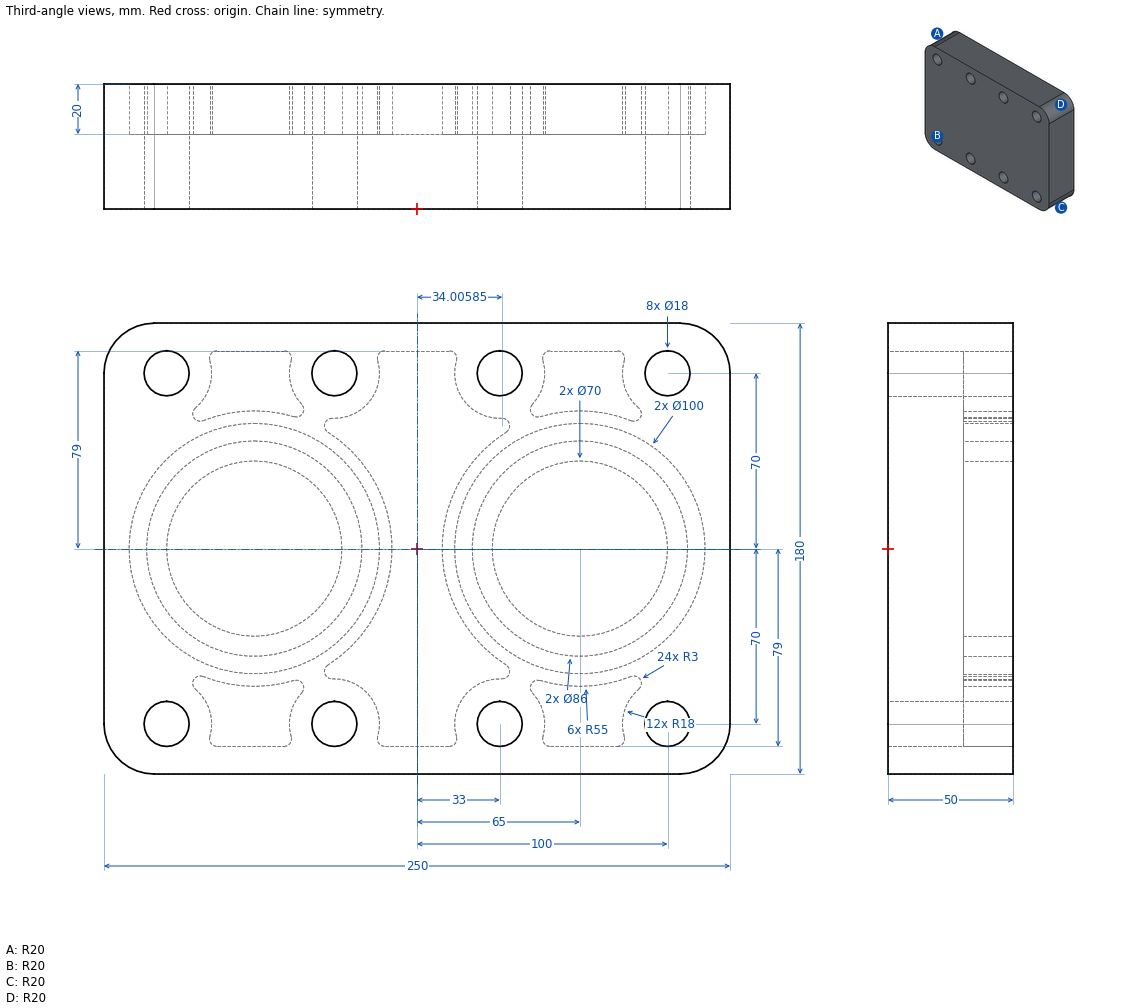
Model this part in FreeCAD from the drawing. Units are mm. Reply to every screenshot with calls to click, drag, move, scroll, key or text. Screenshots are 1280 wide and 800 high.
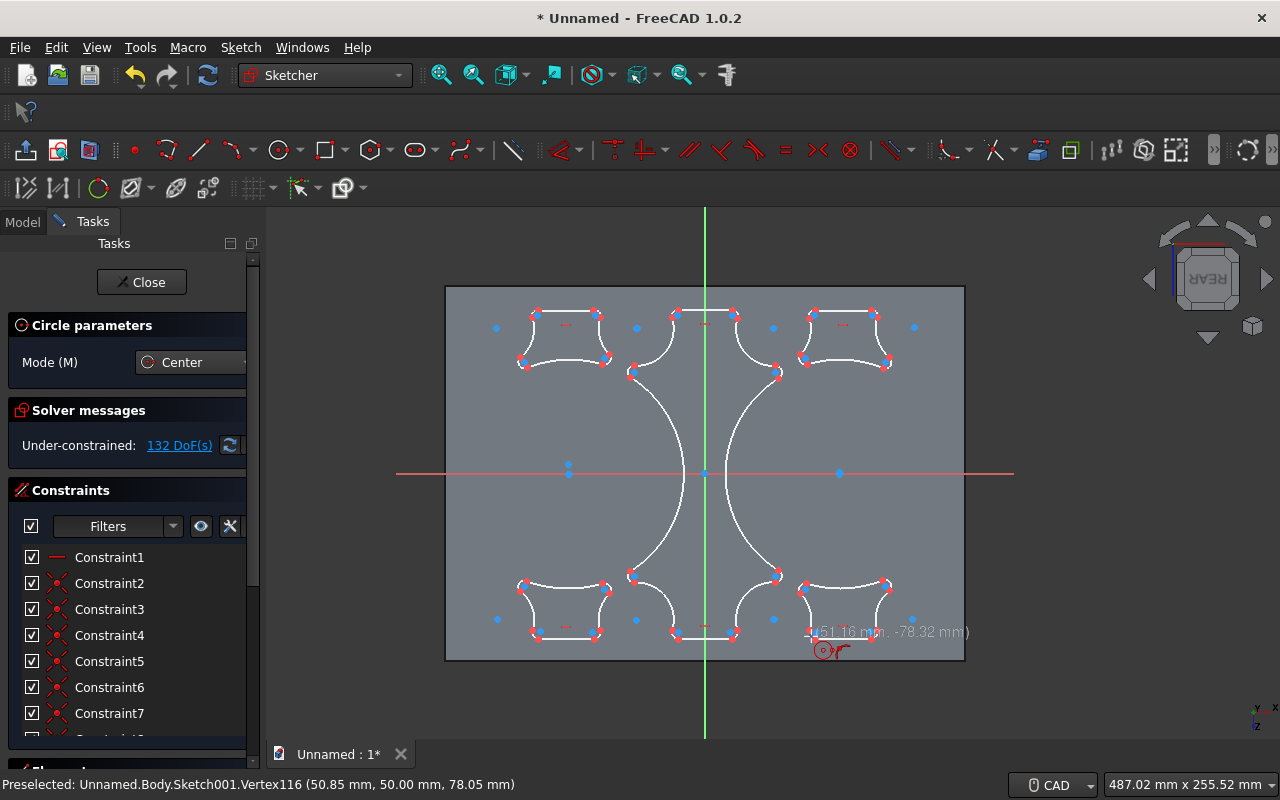
click(840, 474)
move(914, 400)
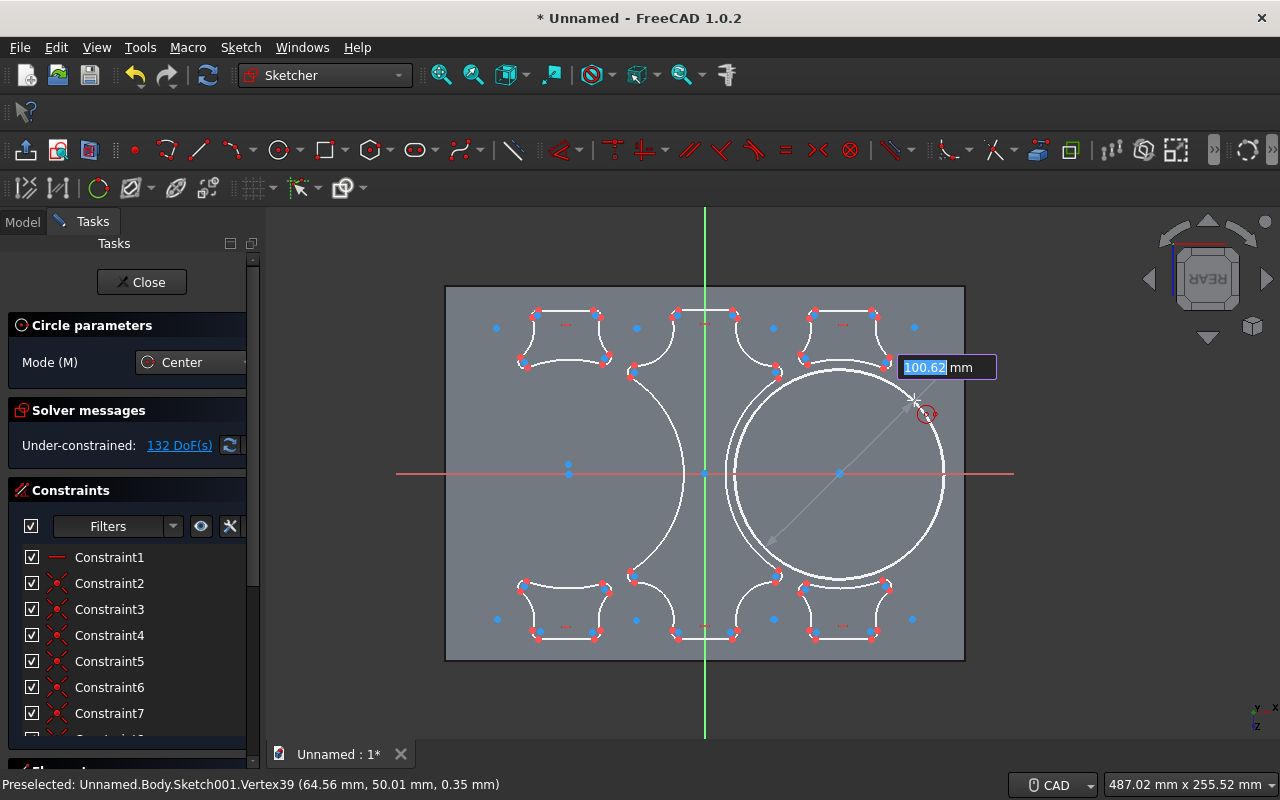
text(100)
key(Return)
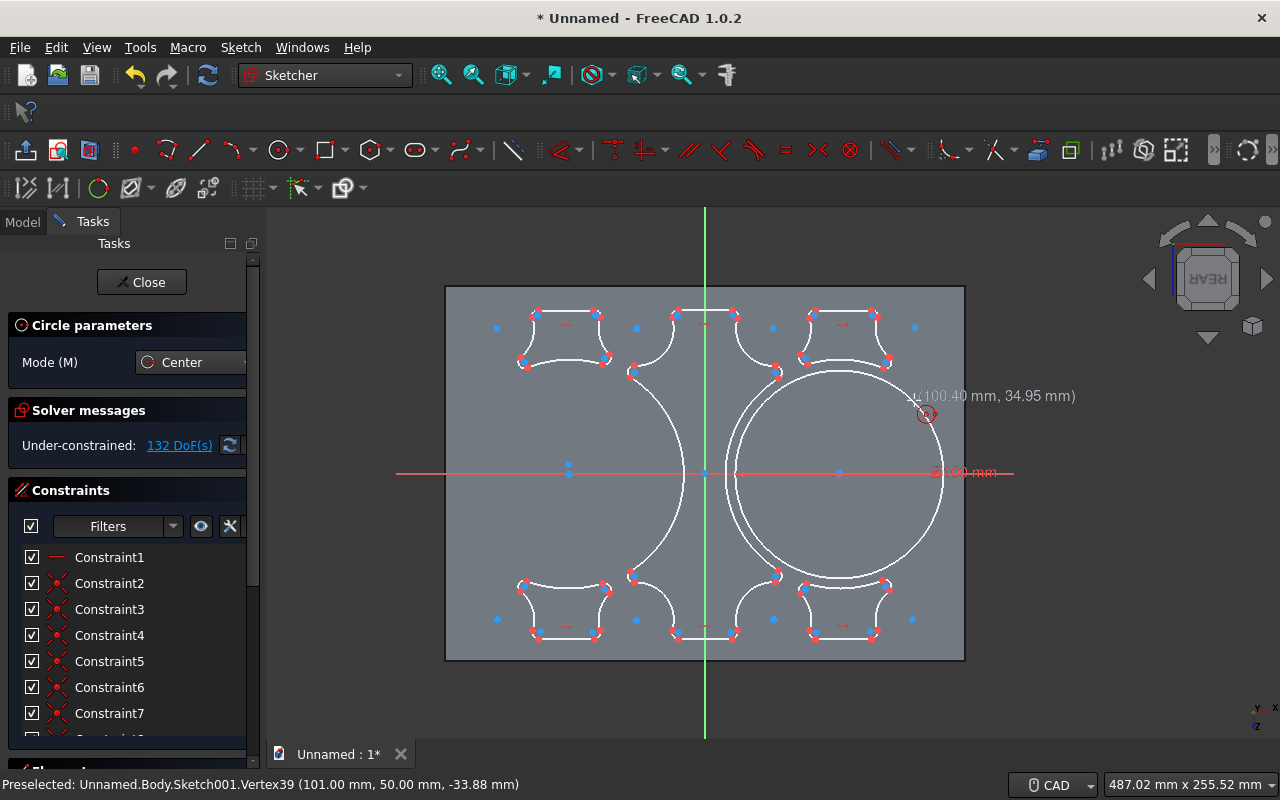
click(840, 474)
move(892, 422)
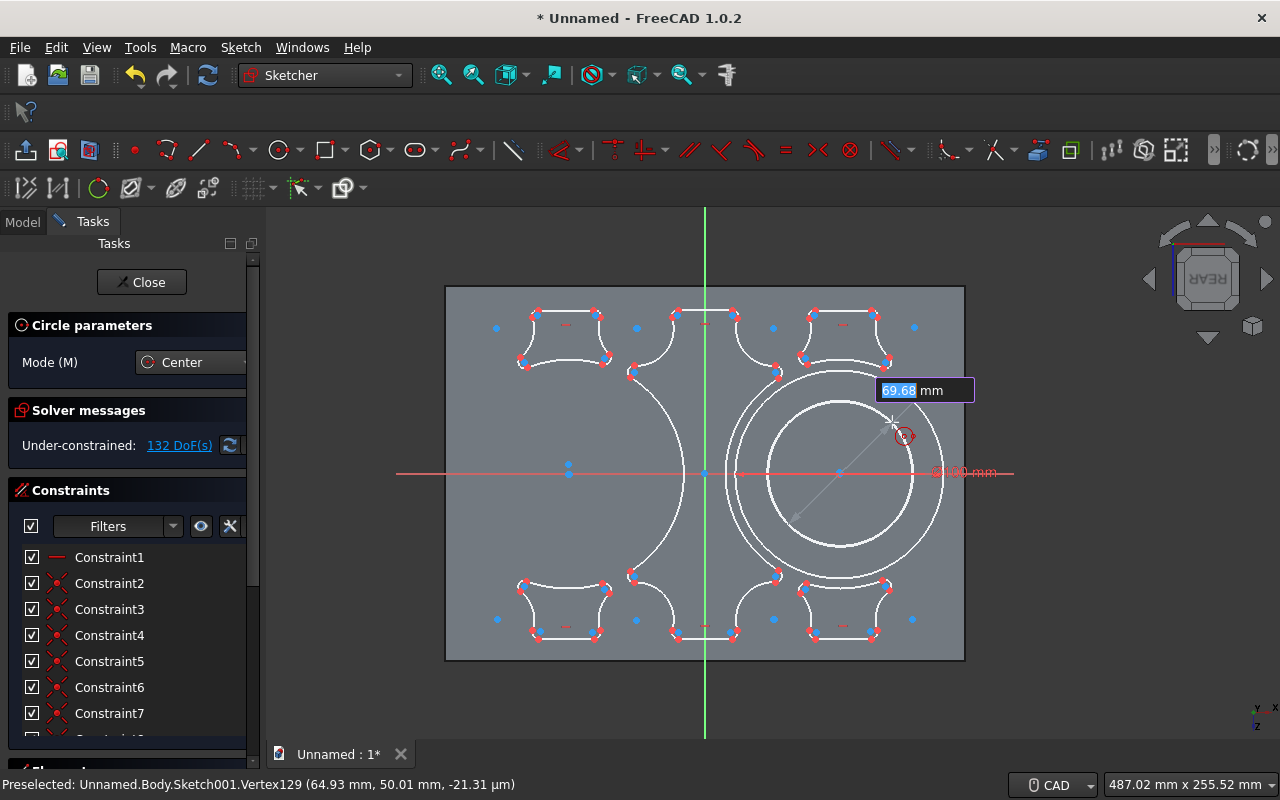
text(70)
key(Return)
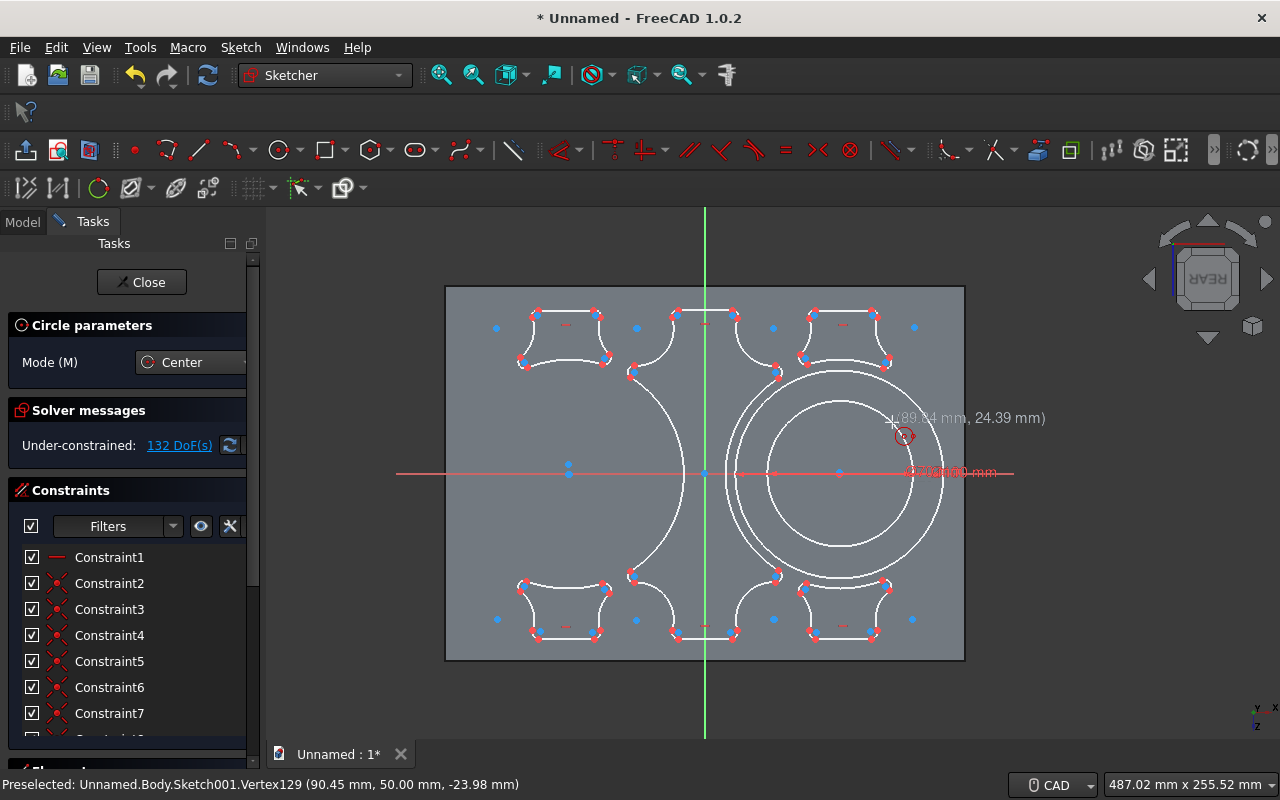
click(570, 474)
move(496, 400)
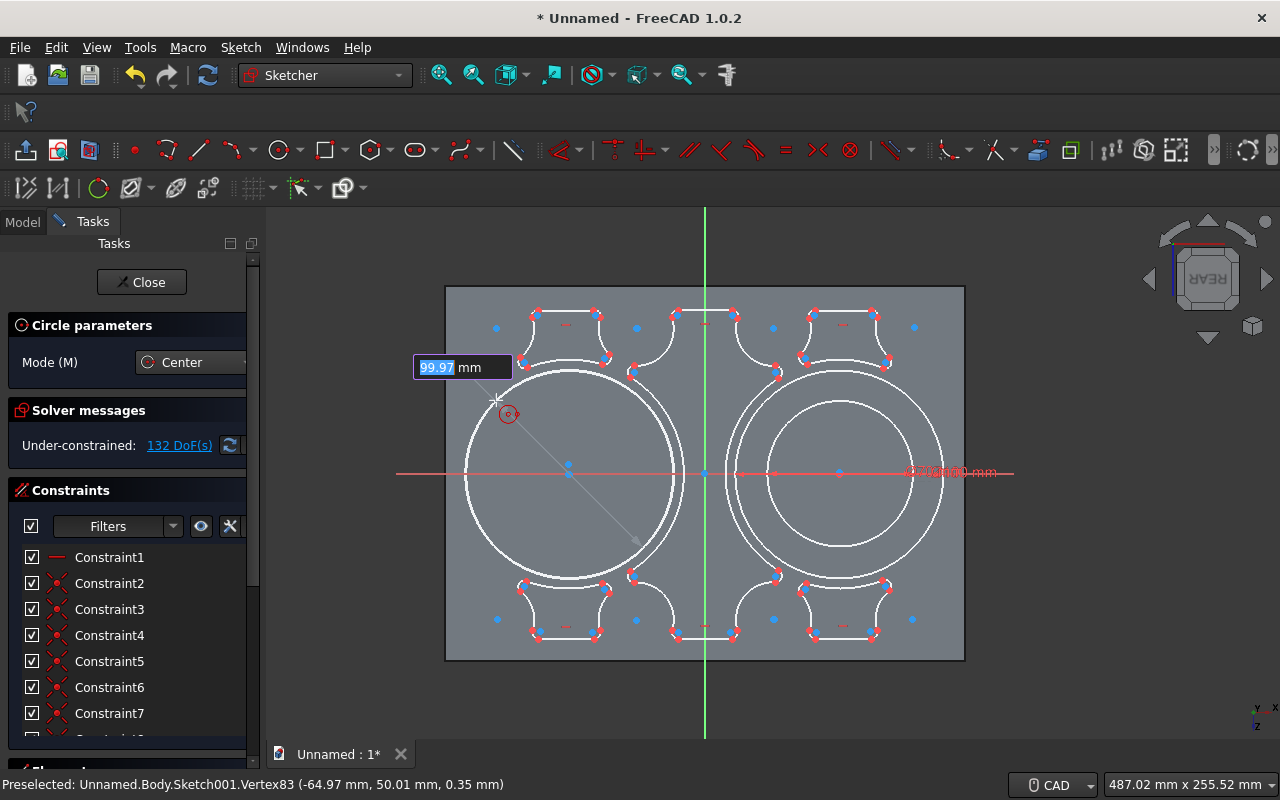
text(100)
key(Return)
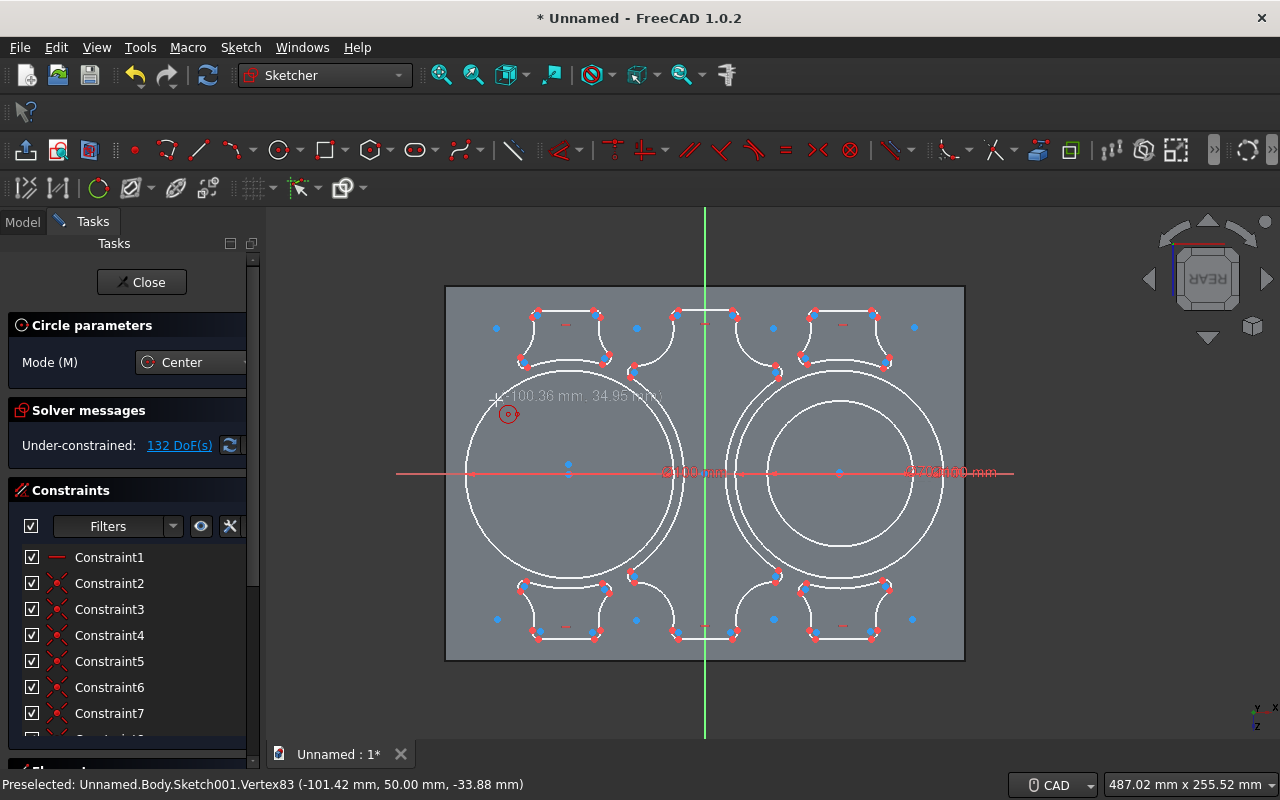
click(570, 474)
move(621, 422)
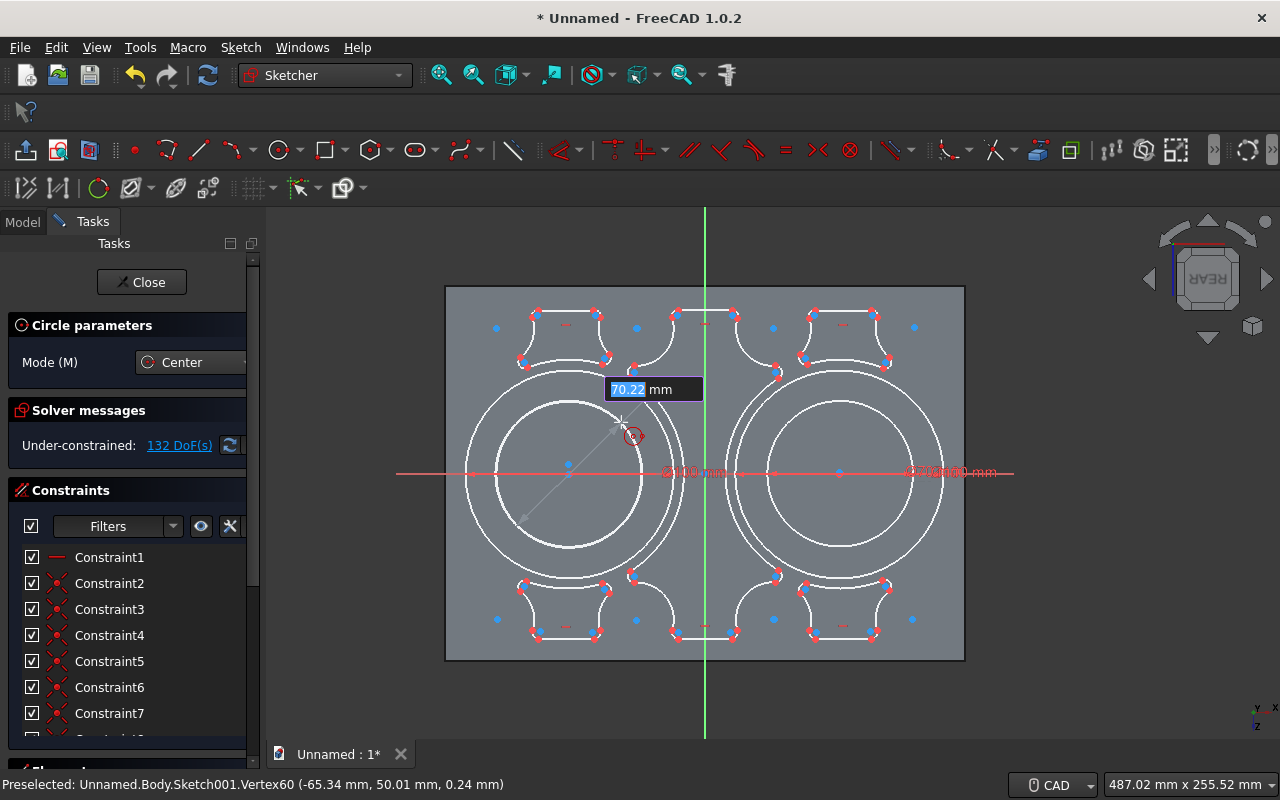
text(70)
key(Return)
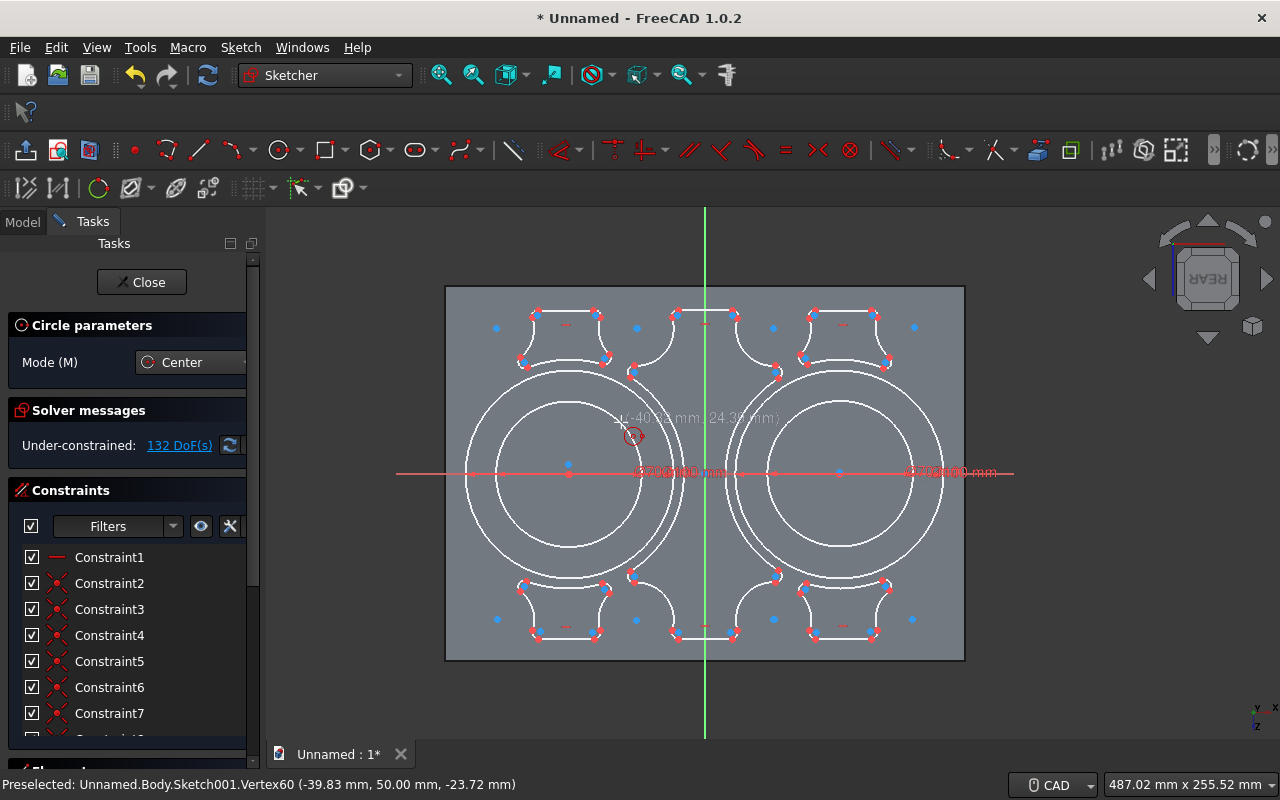
click(840, 474)
move(904, 410)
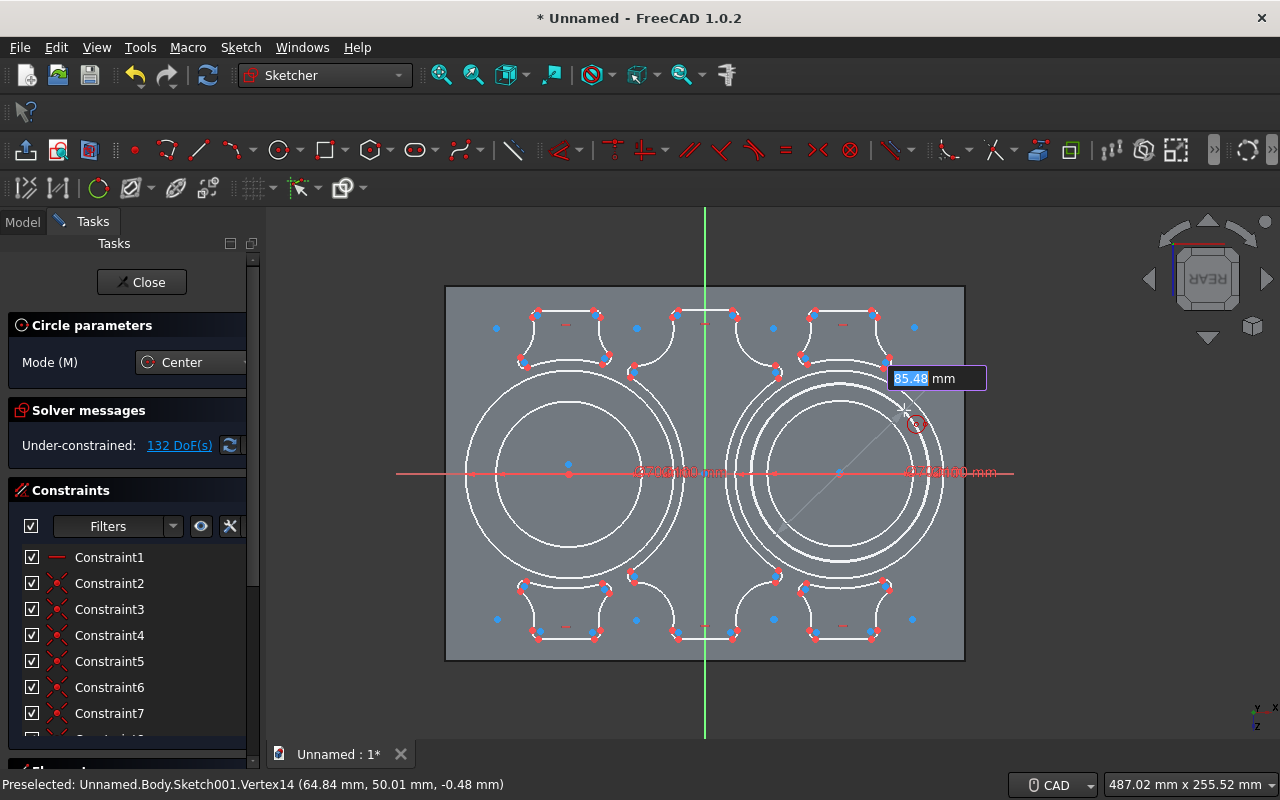
text(86)
key(Return)